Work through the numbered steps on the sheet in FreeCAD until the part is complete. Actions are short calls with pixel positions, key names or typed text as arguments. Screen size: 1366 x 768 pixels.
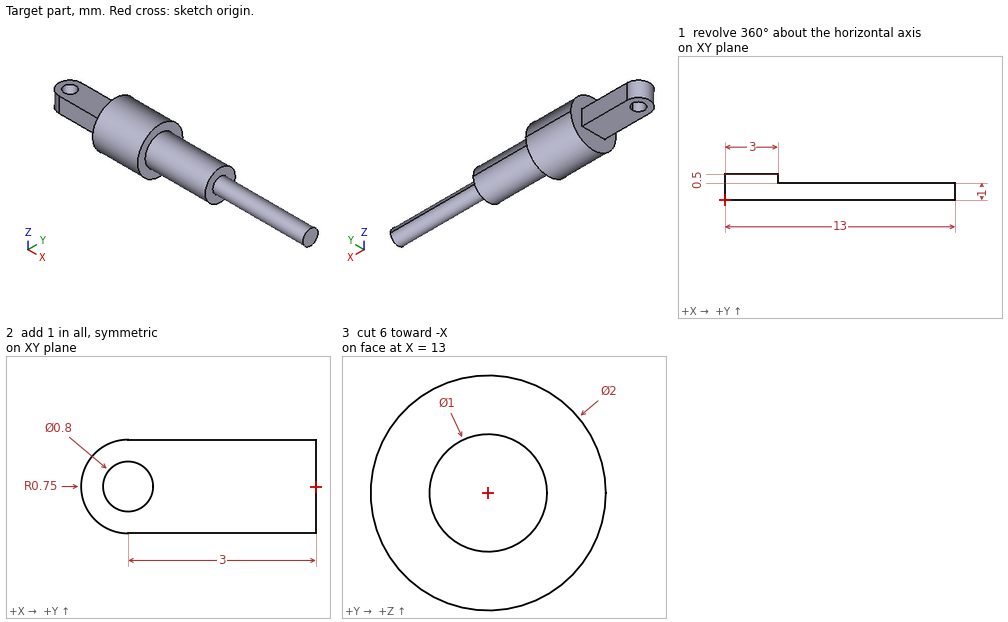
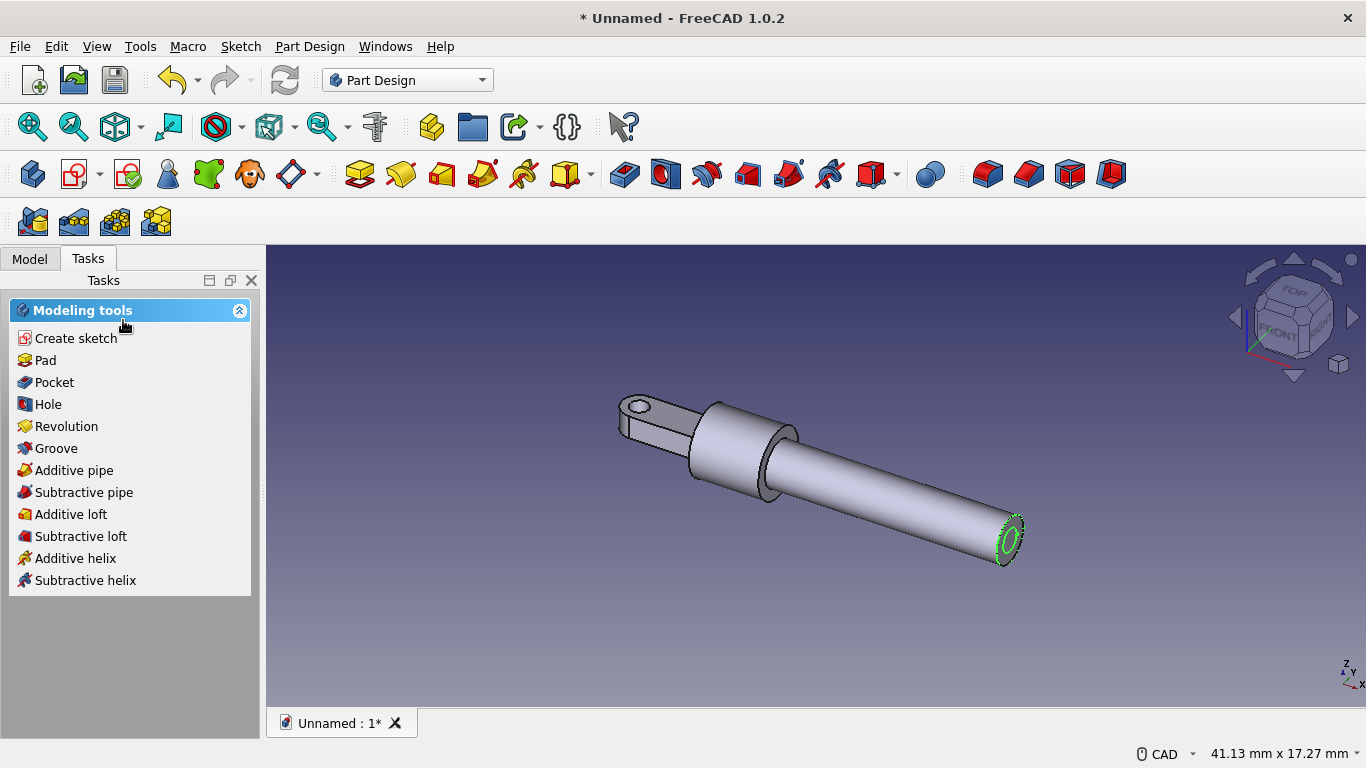
click(625, 174)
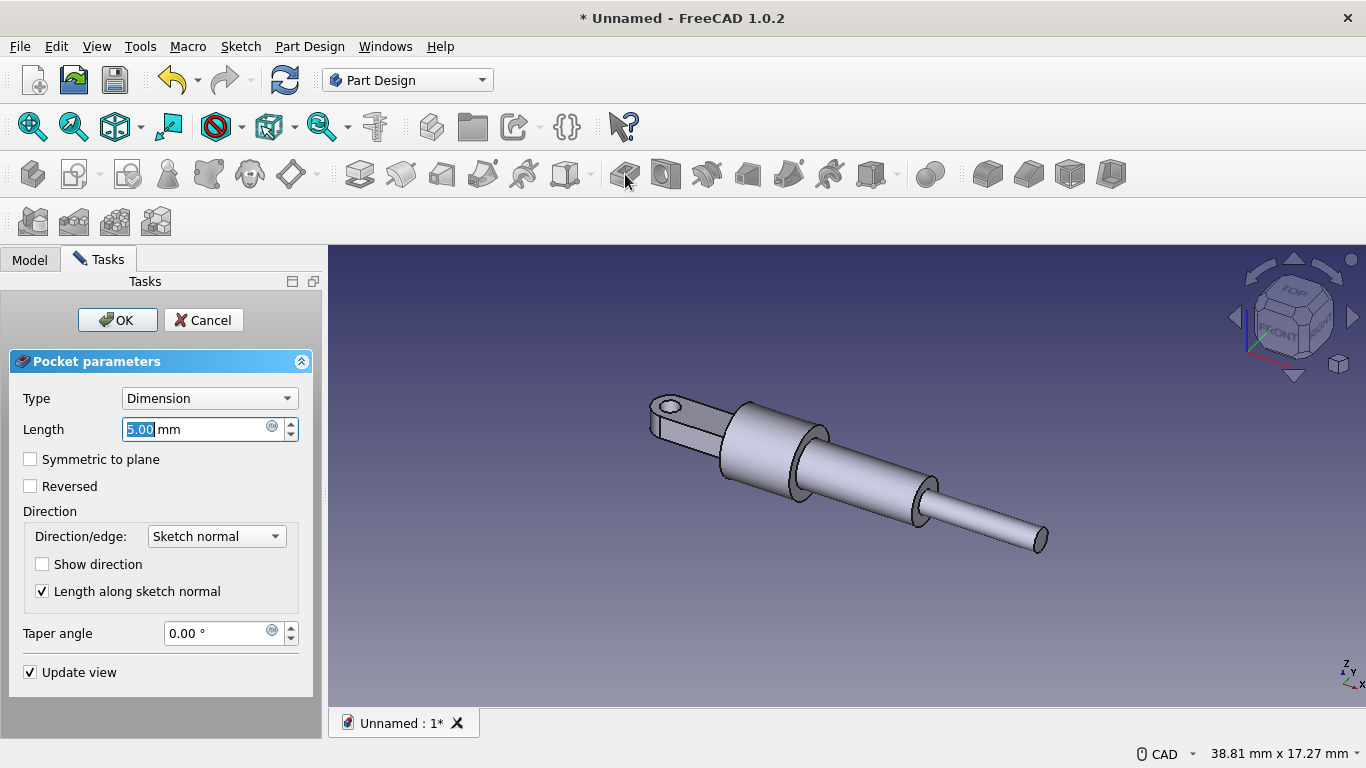
text(6)
key(Tab)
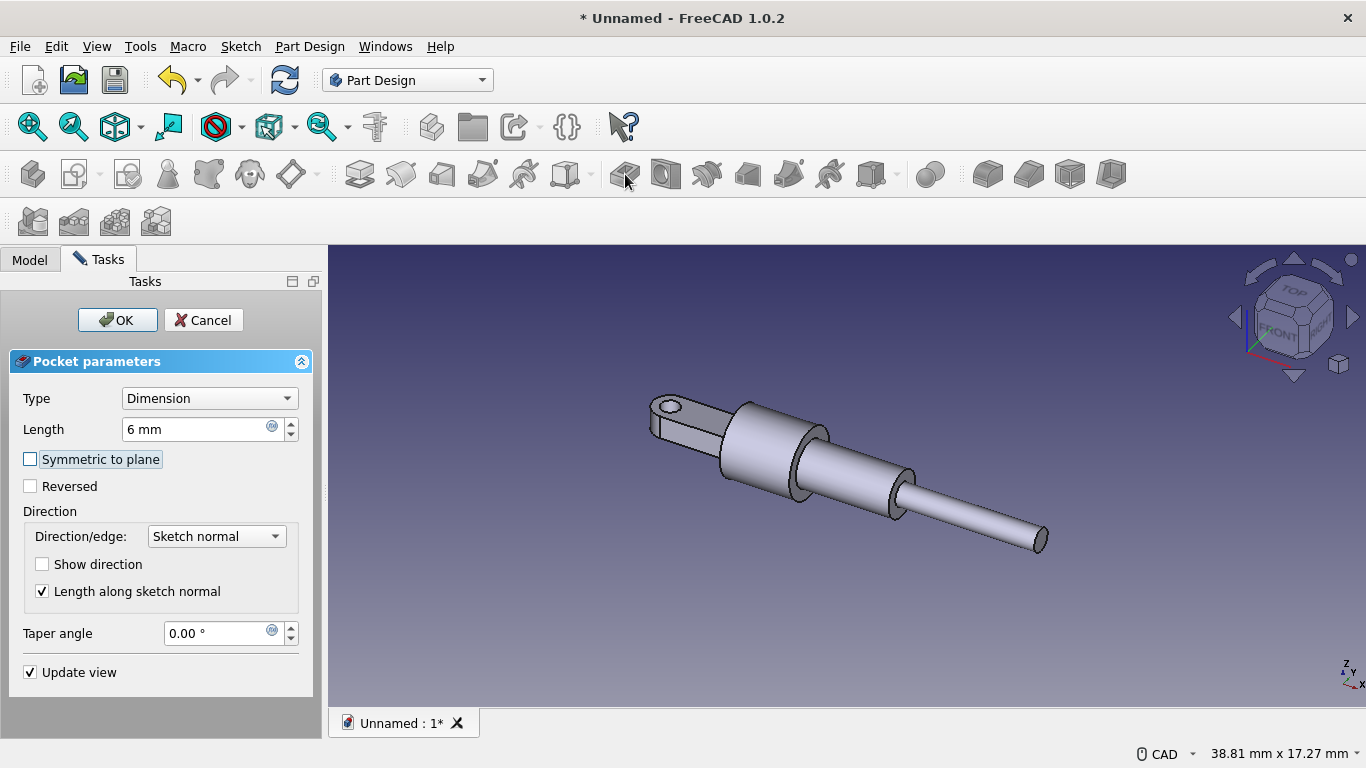
click(118, 320)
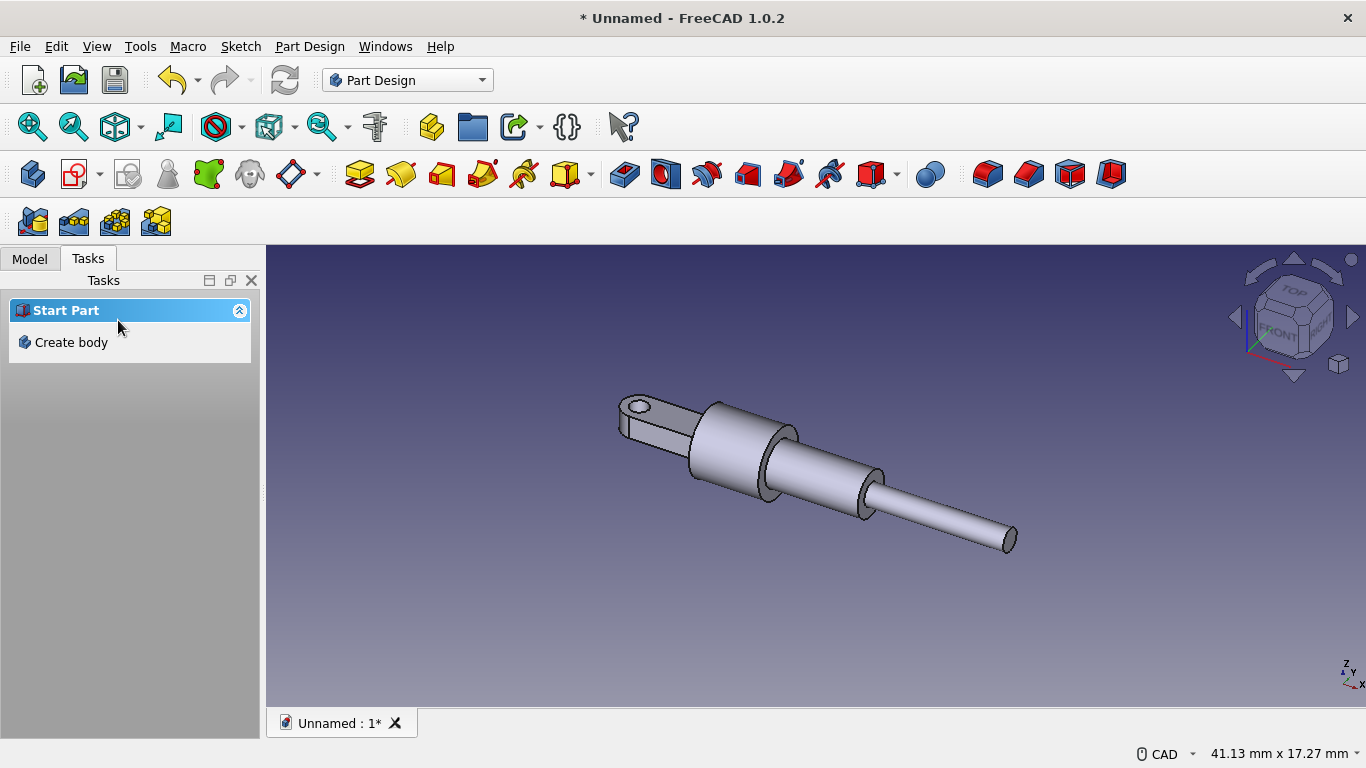
key(0)